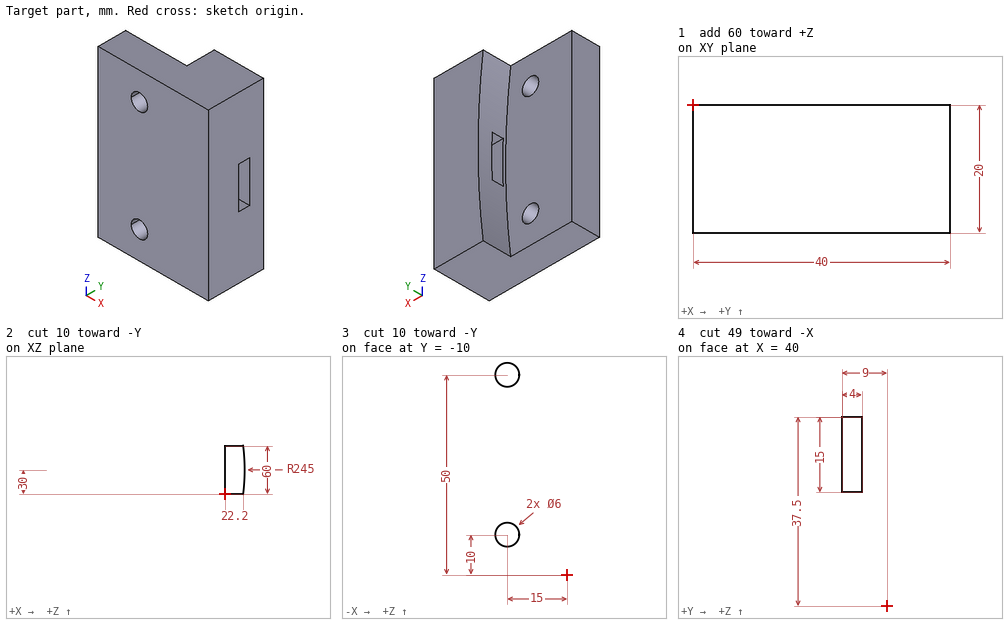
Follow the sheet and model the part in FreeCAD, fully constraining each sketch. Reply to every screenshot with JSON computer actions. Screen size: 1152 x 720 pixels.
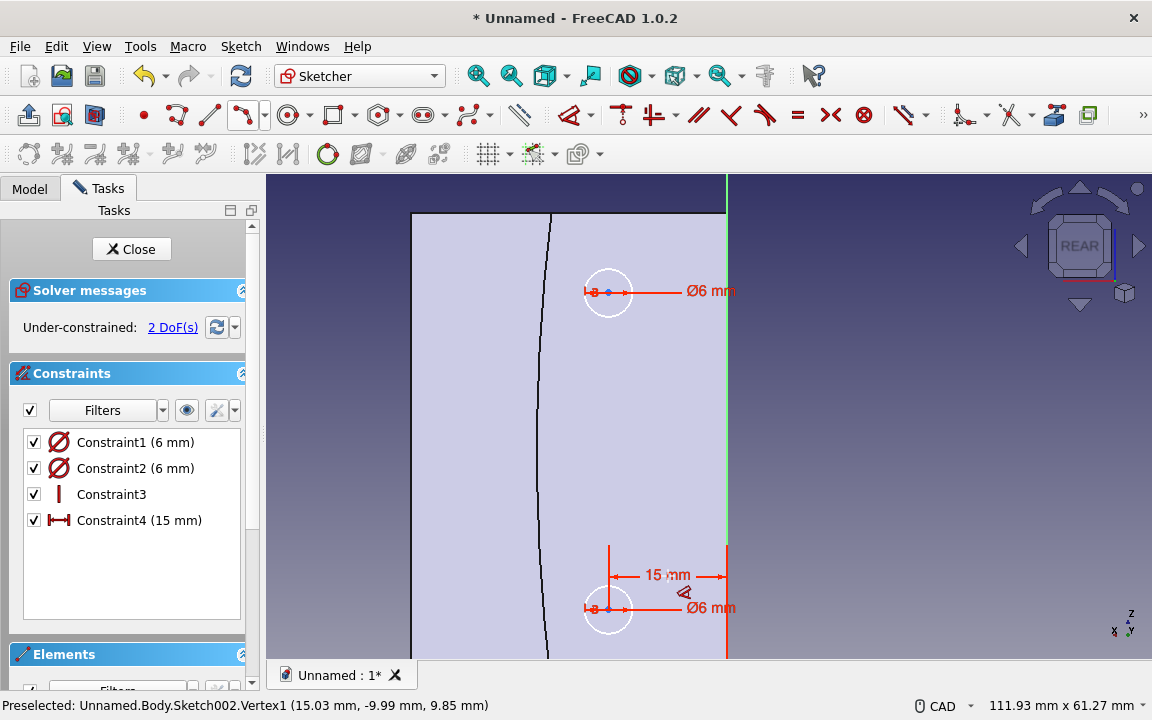
{"action": "left_click", "coordinate": [609, 610]}
{"action": "left_click", "coordinate": [761, 620]}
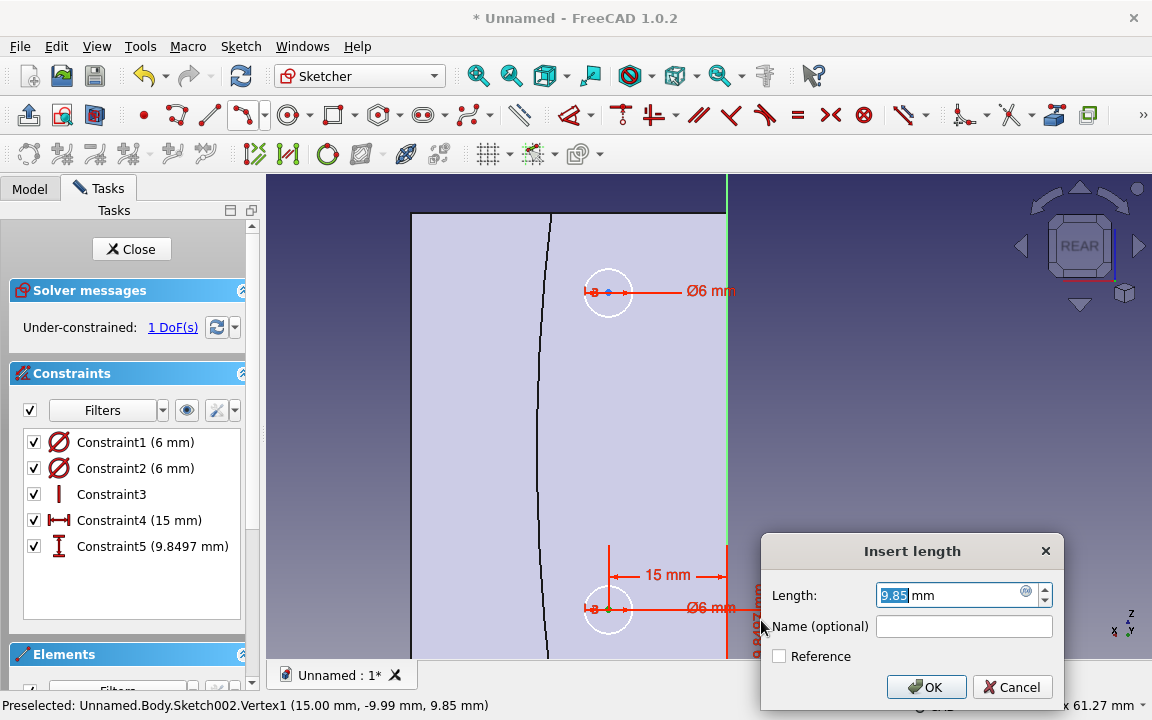
{"action": "type", "text": "10"}
{"action": "key", "text": "Return"}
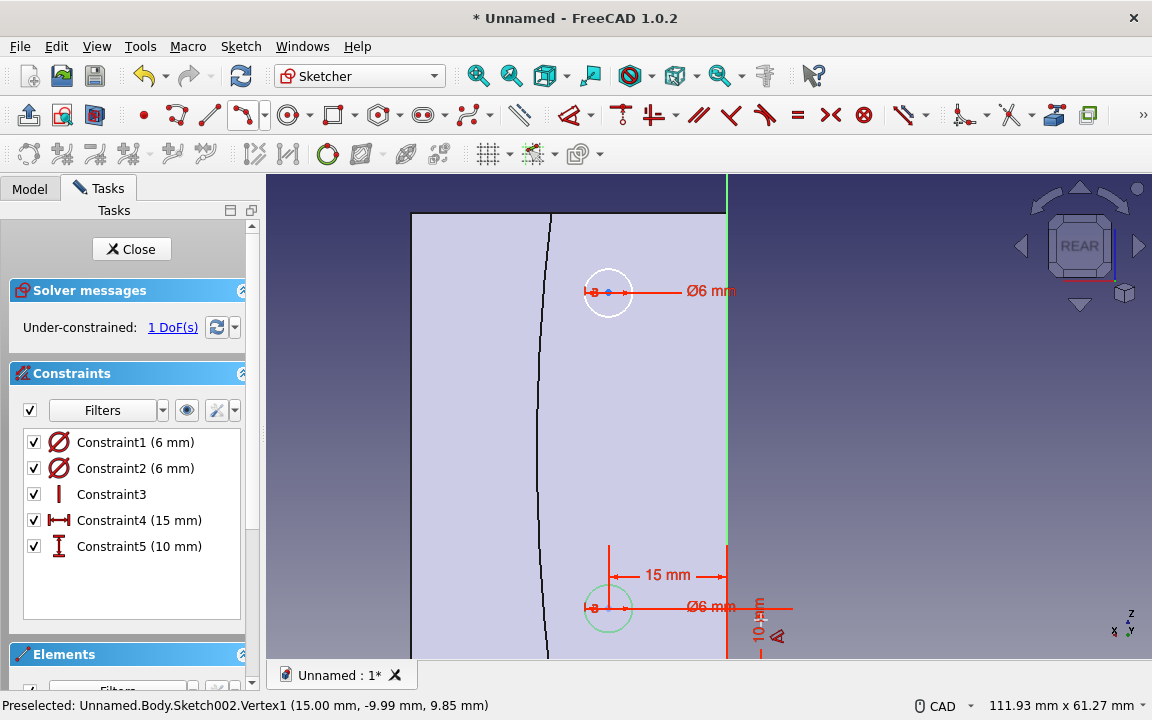
{"action": "left_click", "coordinate": [609, 293]}
{"action": "left_click", "coordinate": [761, 462]}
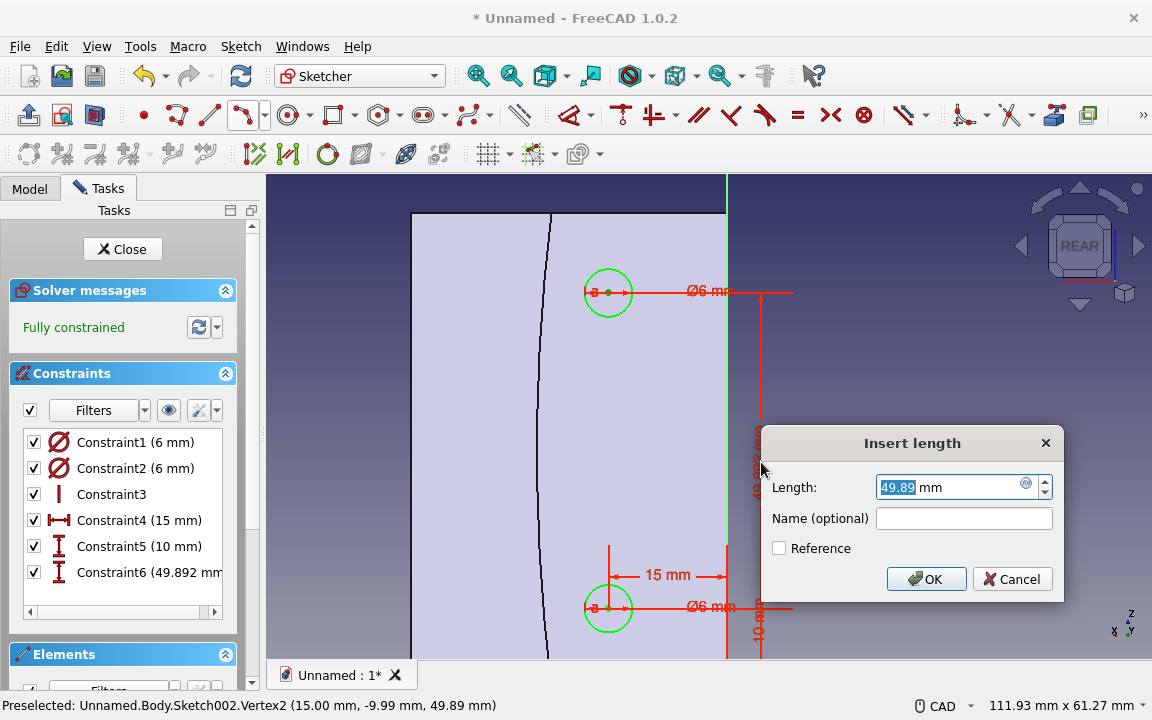
{"action": "type", "text": "50"}
{"action": "key", "text": "Return"}
{"action": "key", "text": "Escape"}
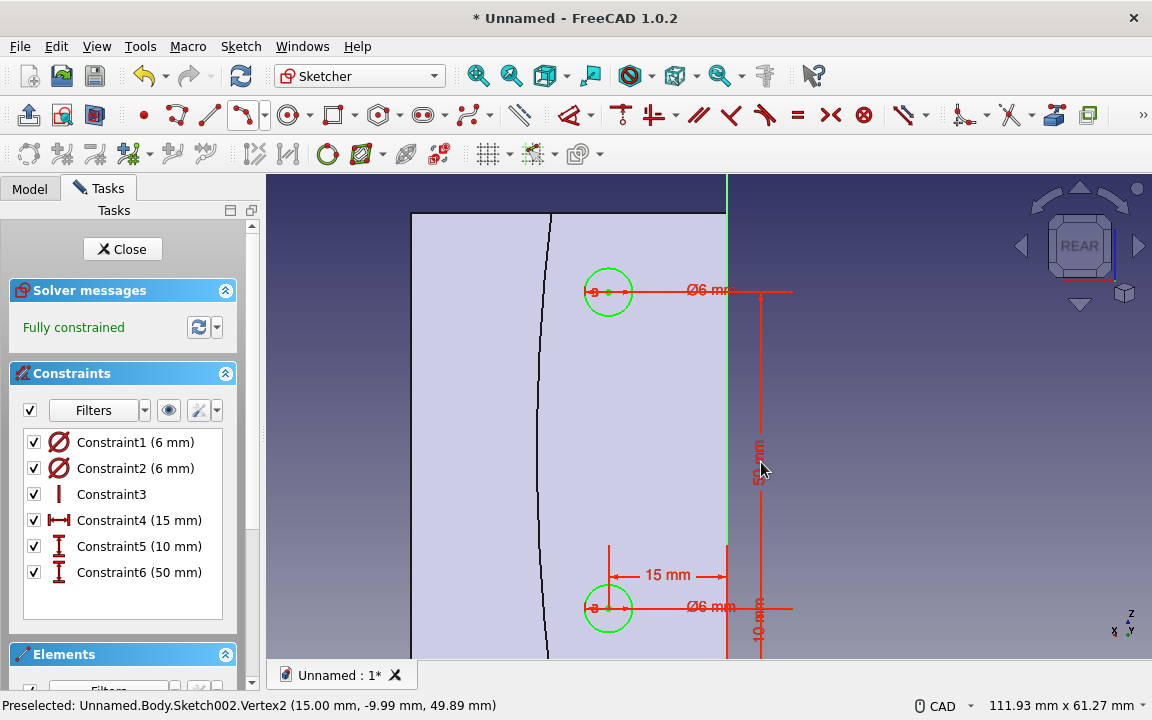
{"action": "left_click", "coordinate": [123, 249]}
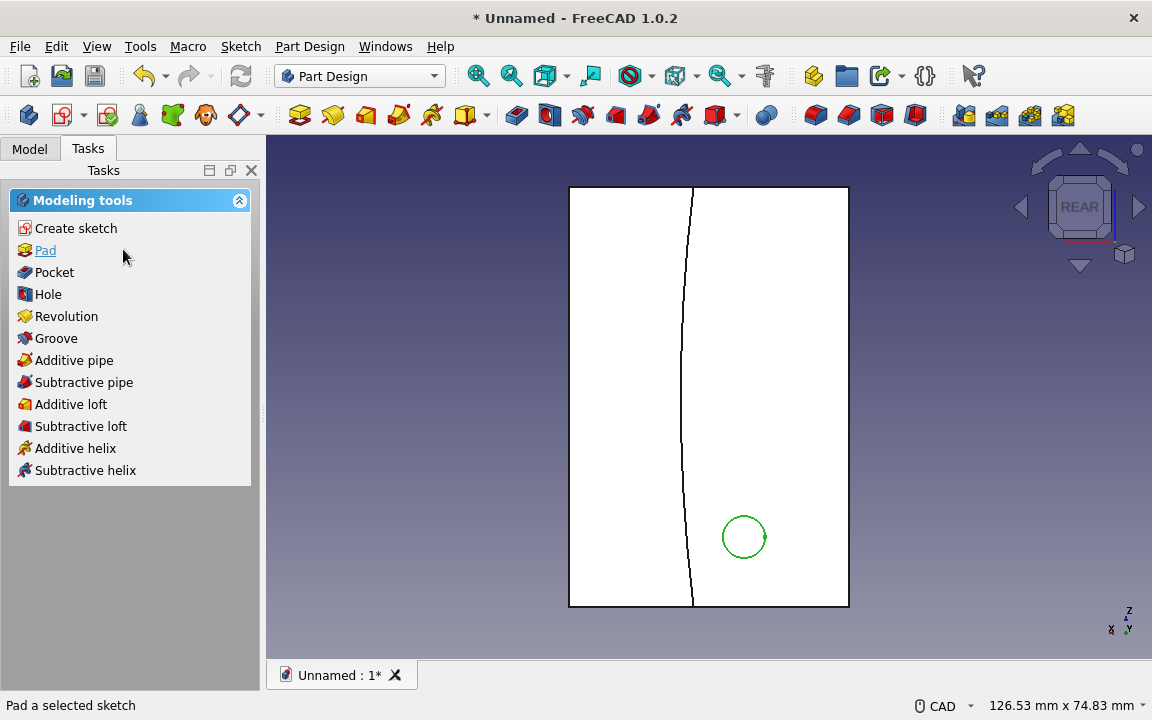
{"action": "left_click", "coordinate": [517, 116]}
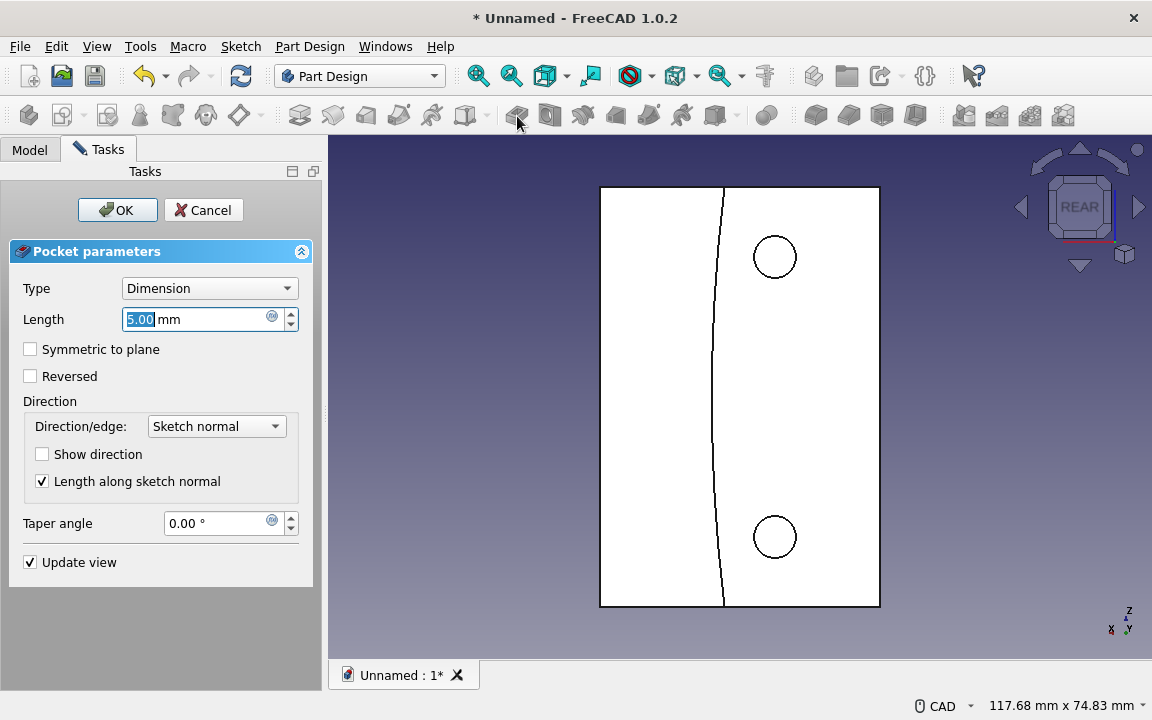
{"action": "type", "text": "10"}
{"action": "key", "text": "Tab"}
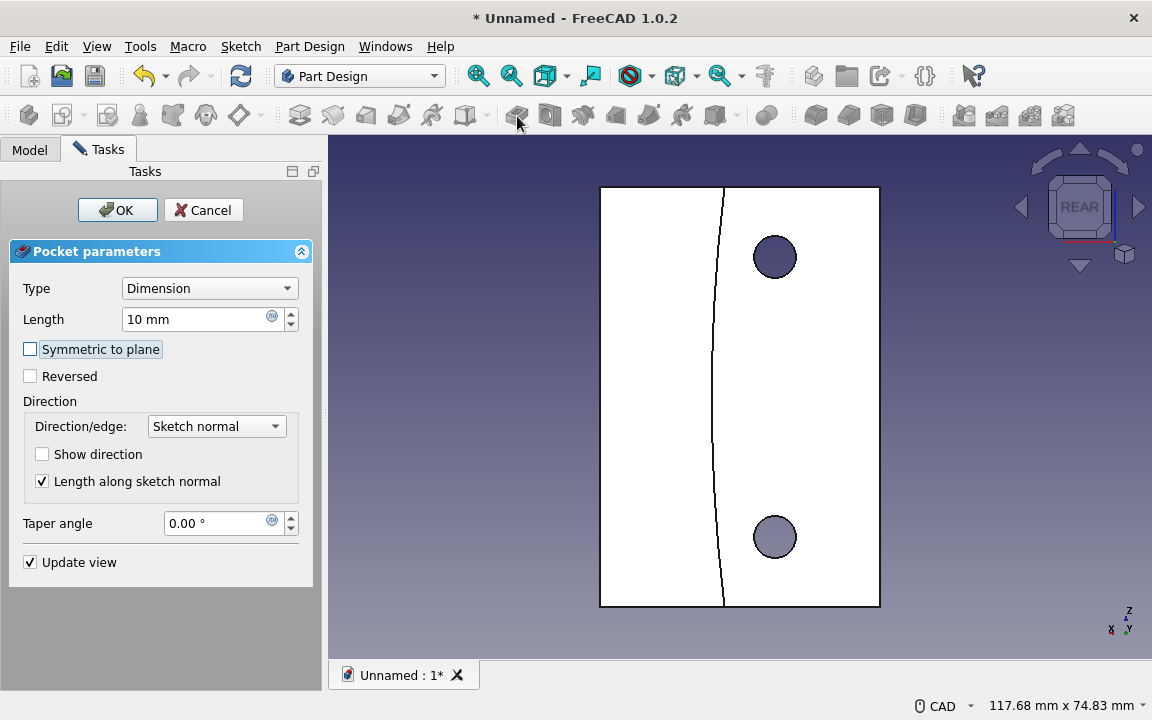
{"action": "left_click", "coordinate": [118, 210]}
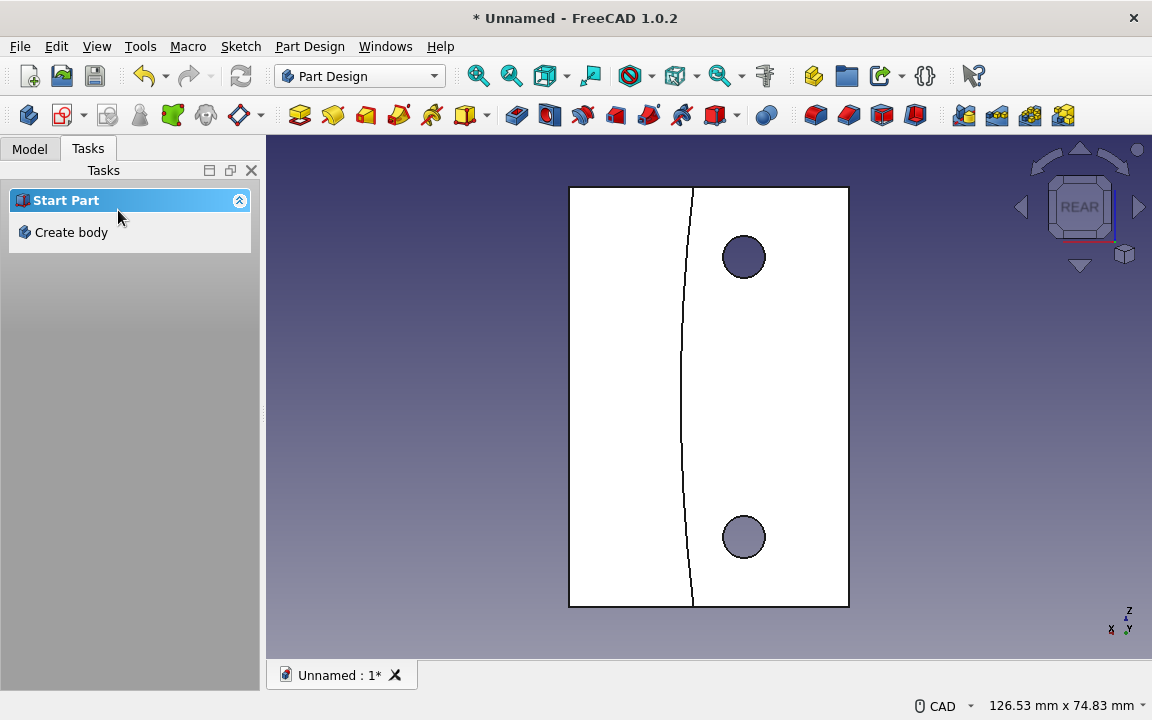
{"action": "key", "text": "0"}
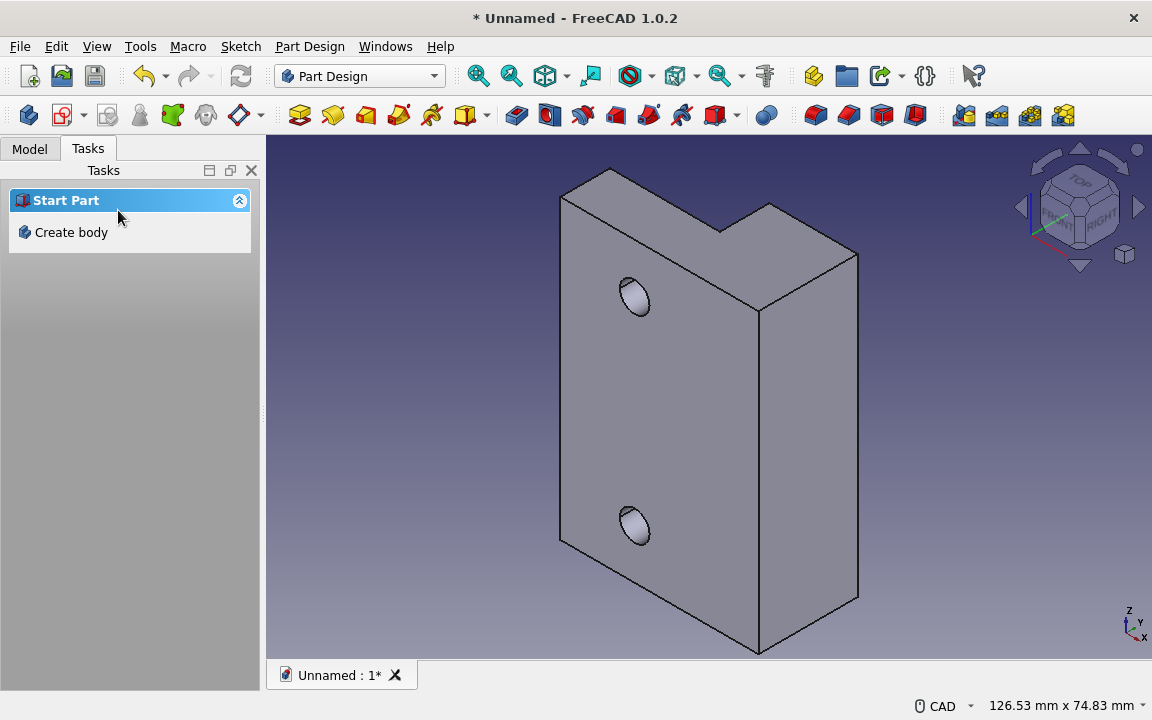
{"action": "left_click", "coordinate": [808, 355]}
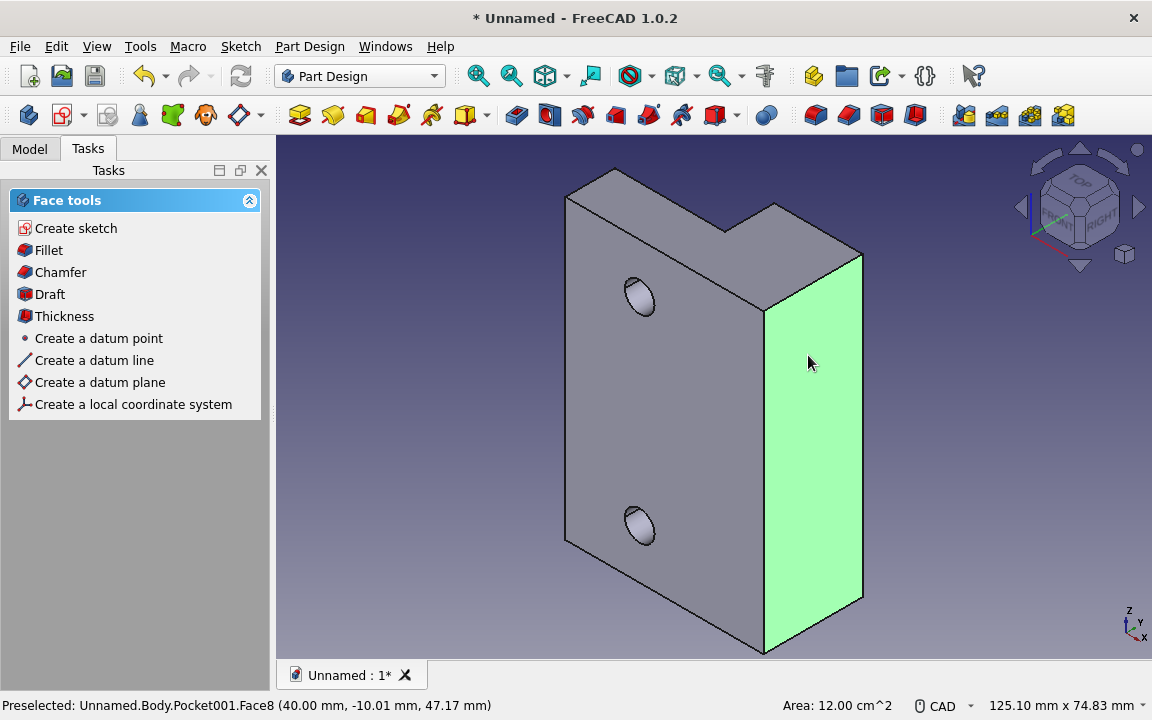
{"action": "left_click", "coordinate": [62, 116]}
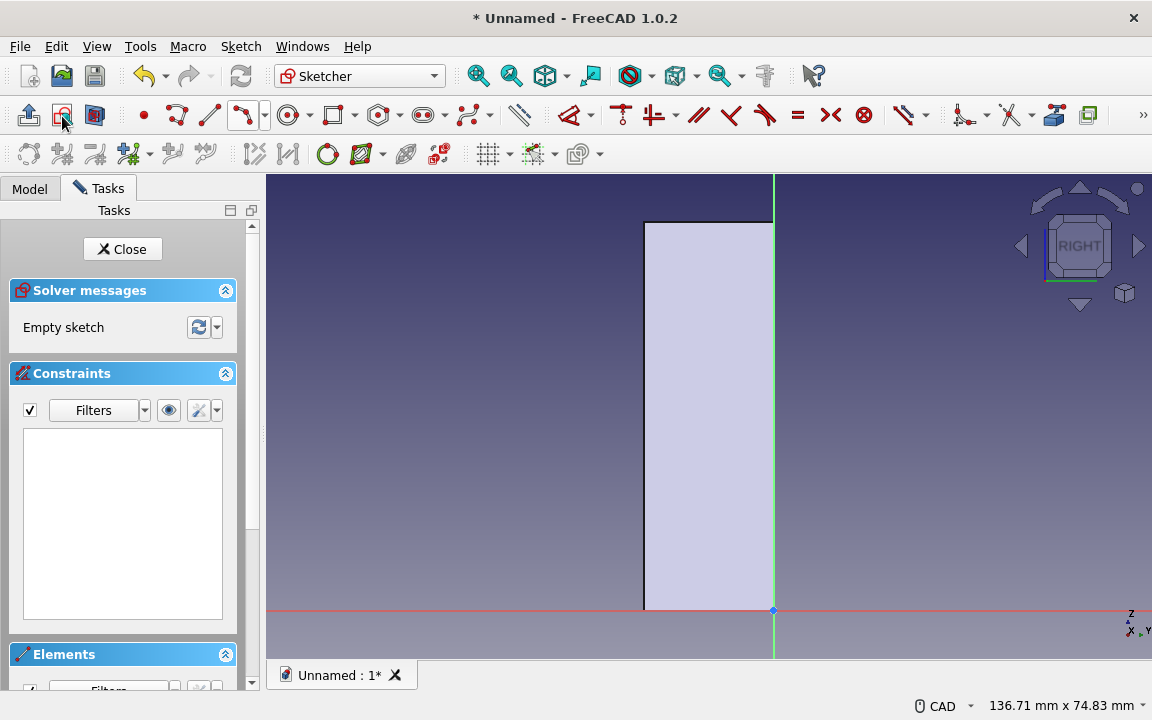
{"action": "scroll", "coordinate": [766, 417], "scroll_direction": "up", "scroll_amount": 6}